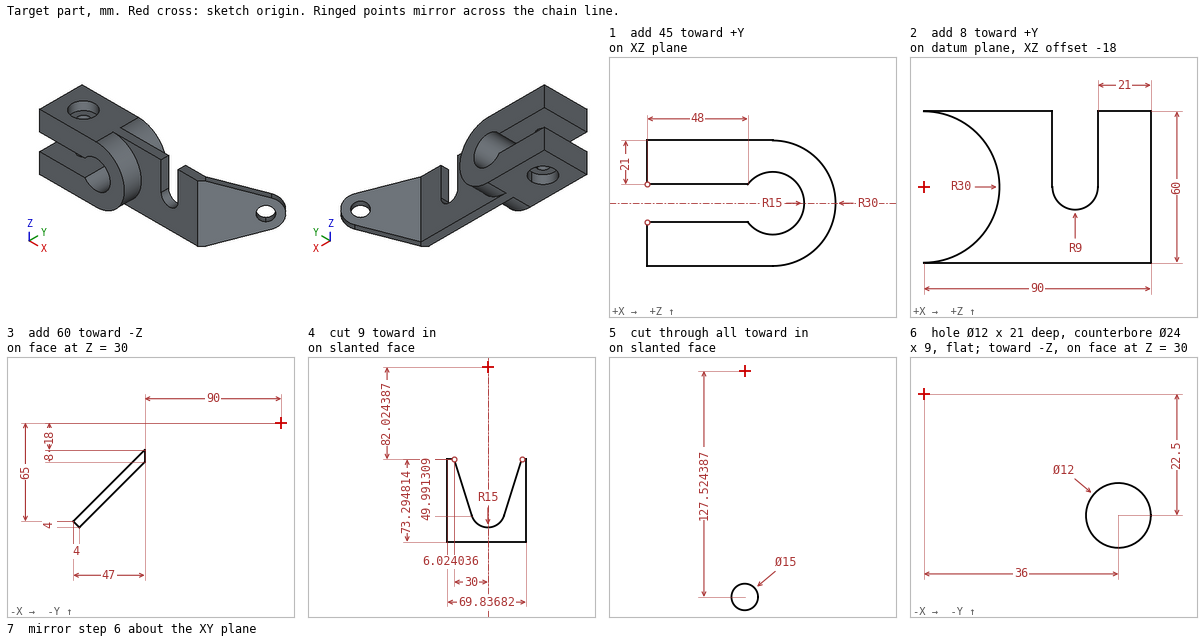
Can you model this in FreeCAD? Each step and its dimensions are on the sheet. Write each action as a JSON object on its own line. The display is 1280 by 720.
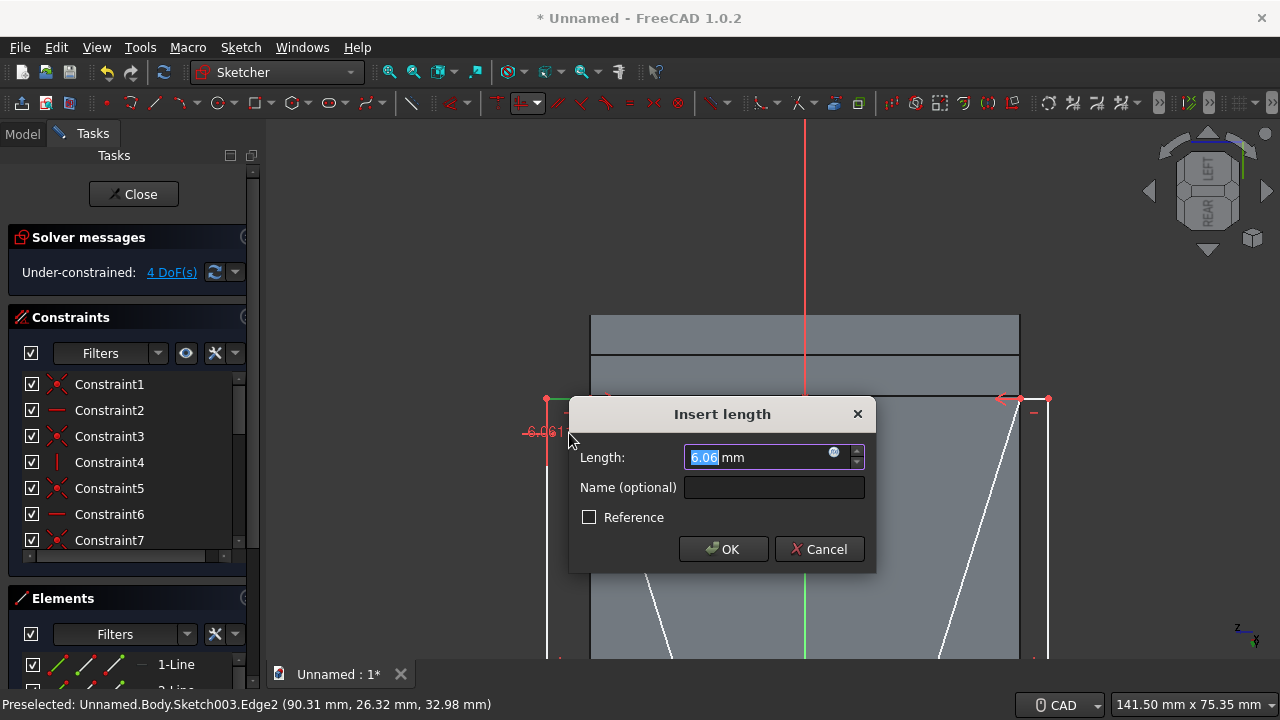
{"action": "type", "text": "6.024036"}
{"action": "key", "text": "Return"}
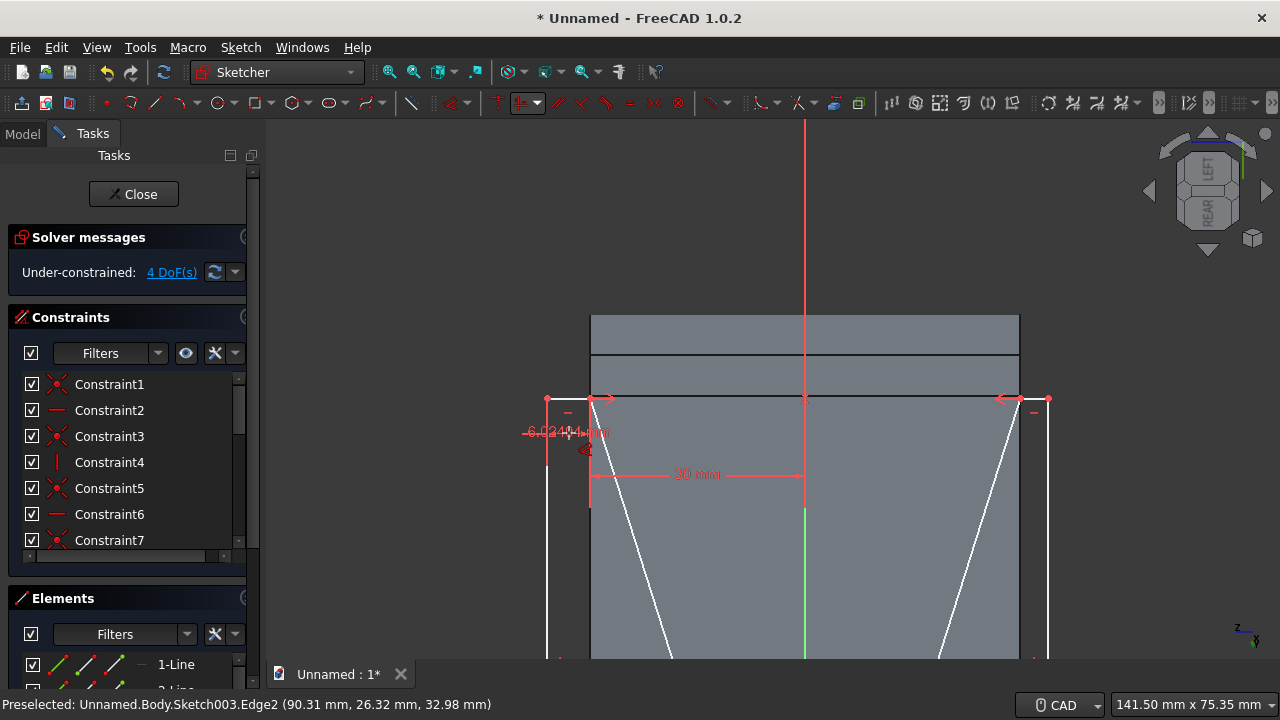
{"action": "scroll", "coordinate": [664, 400], "scroll_direction": "down", "scroll_amount": 6}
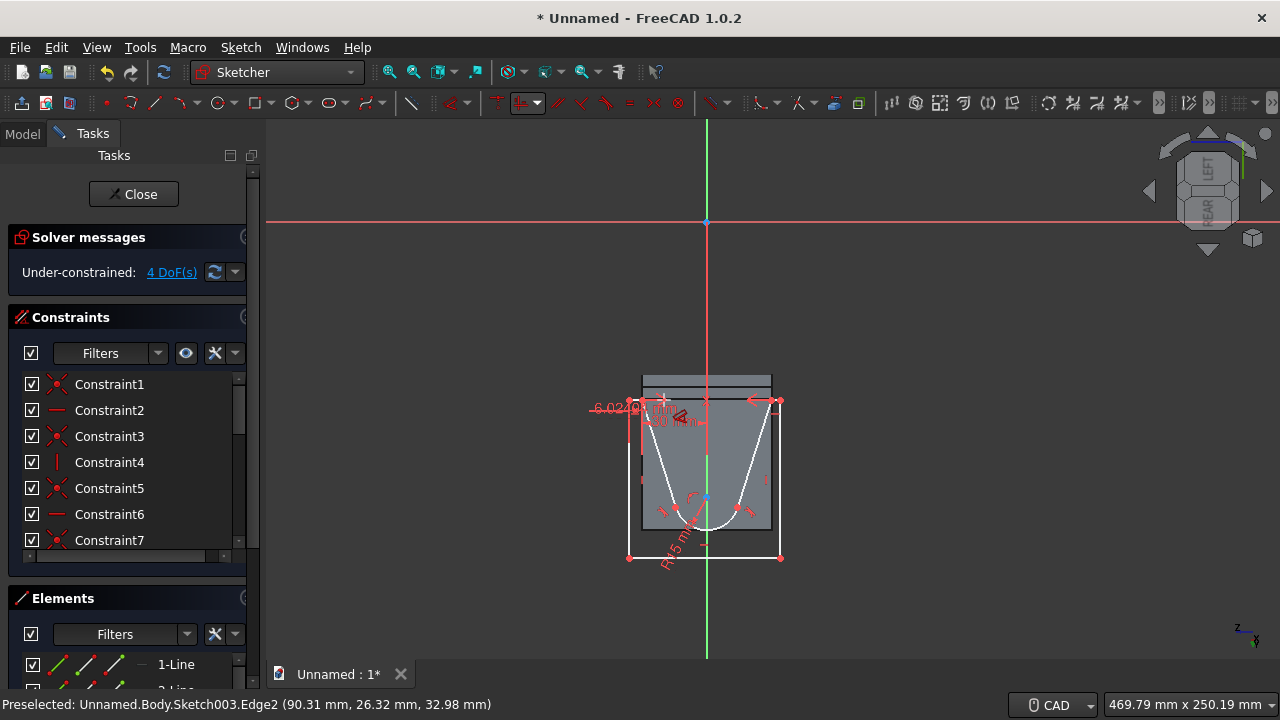
{"action": "left_click", "coordinate": [674, 558]}
{"action": "left_click", "coordinate": [670, 592]}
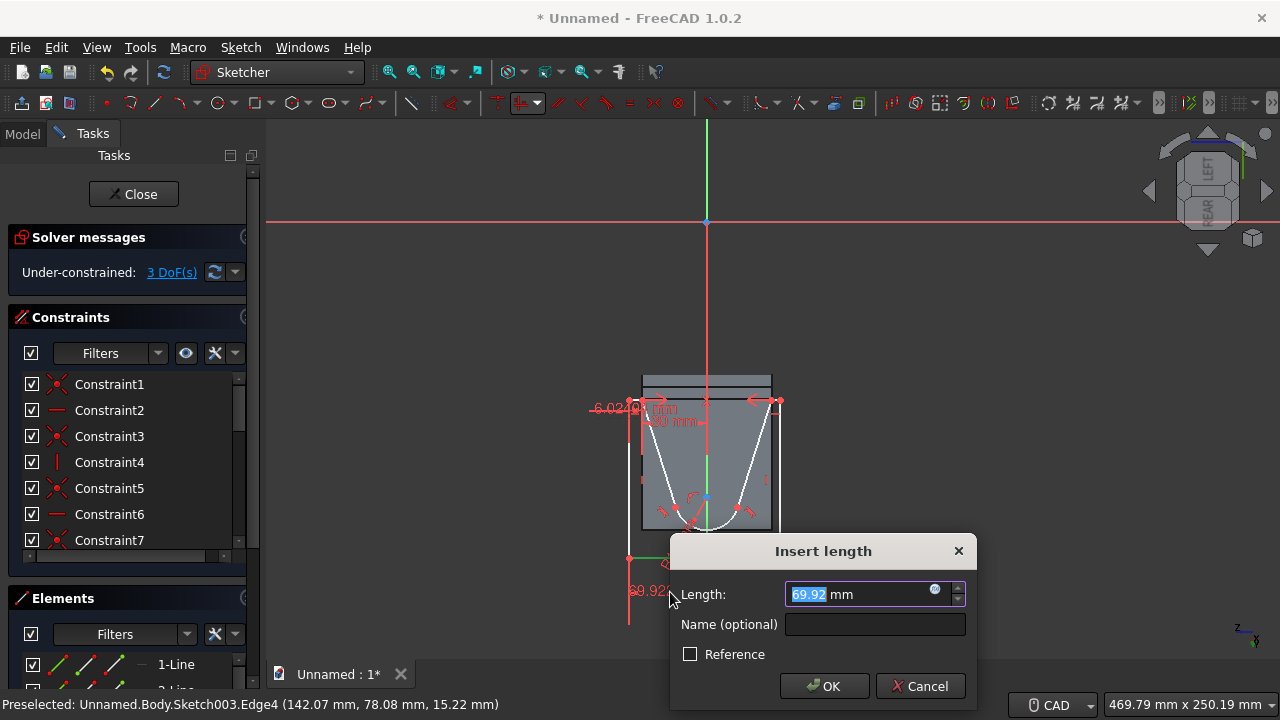
{"action": "type", "text": "69.83682"}
{"action": "key", "text": "Return"}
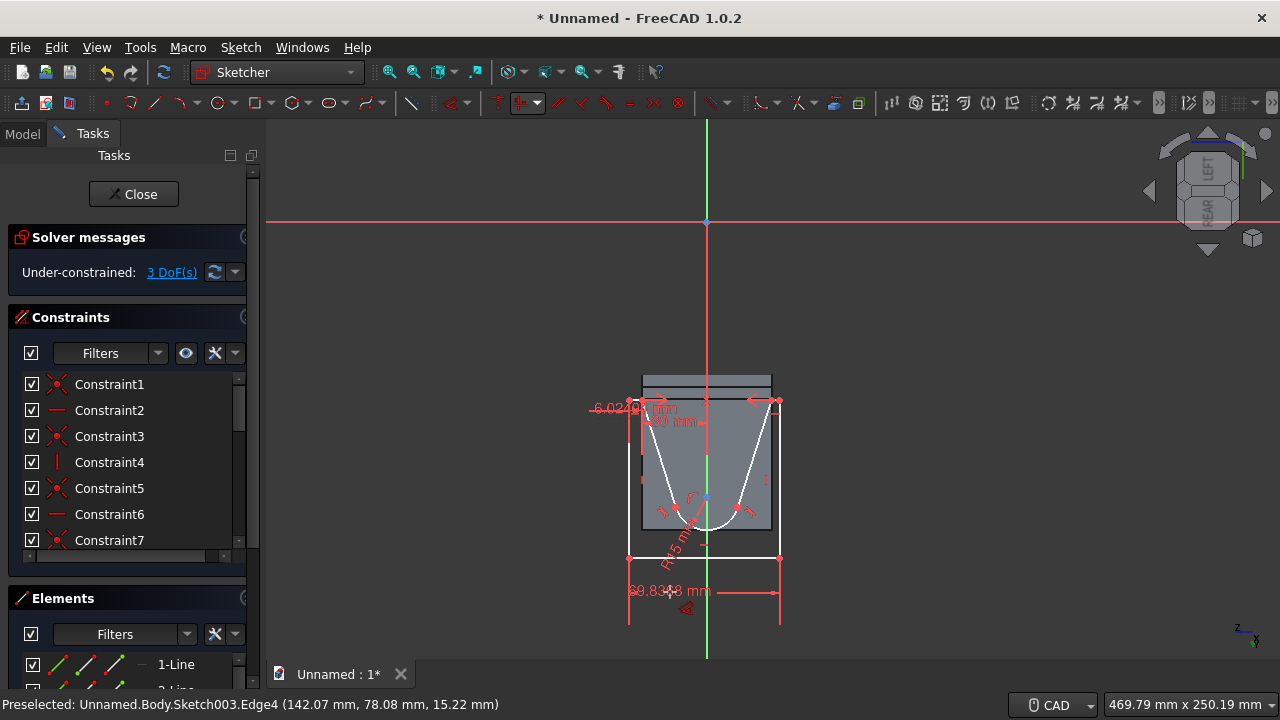
{"action": "left_click", "coordinate": [629, 447]}
{"action": "left_click", "coordinate": [595, 479]}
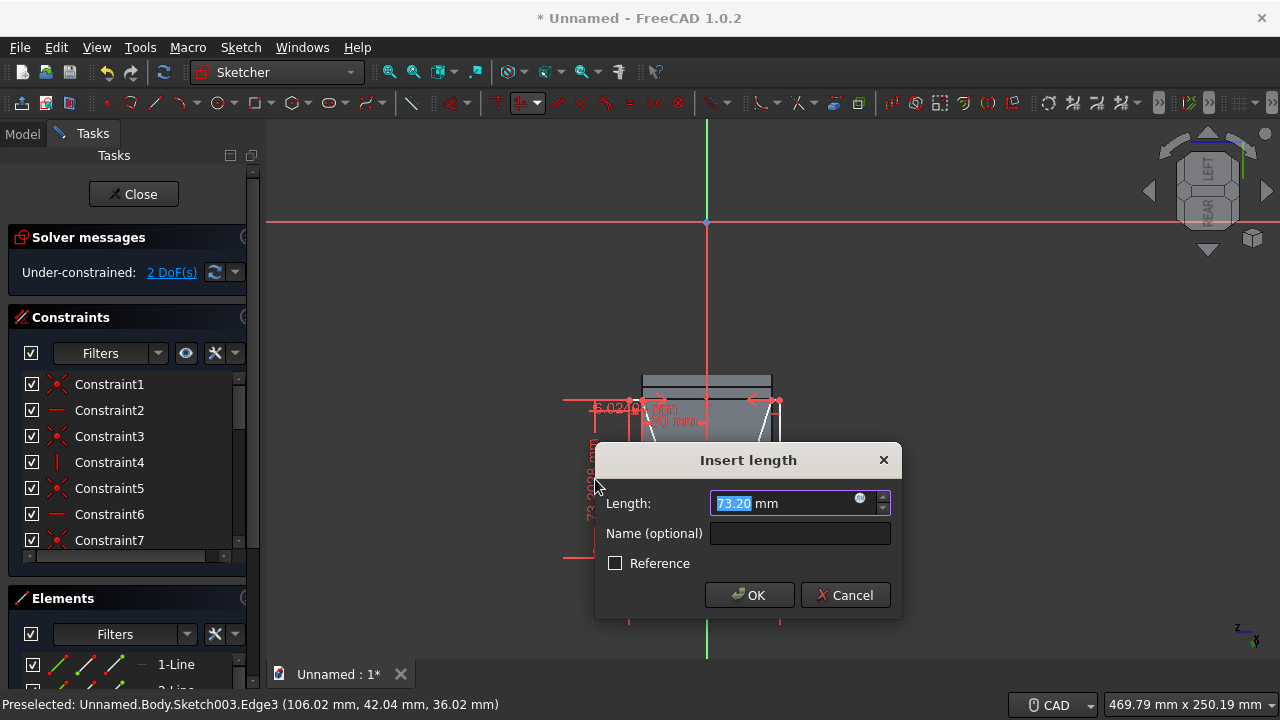
{"action": "type", "text": "73.294814"}
{"action": "key", "text": "Return"}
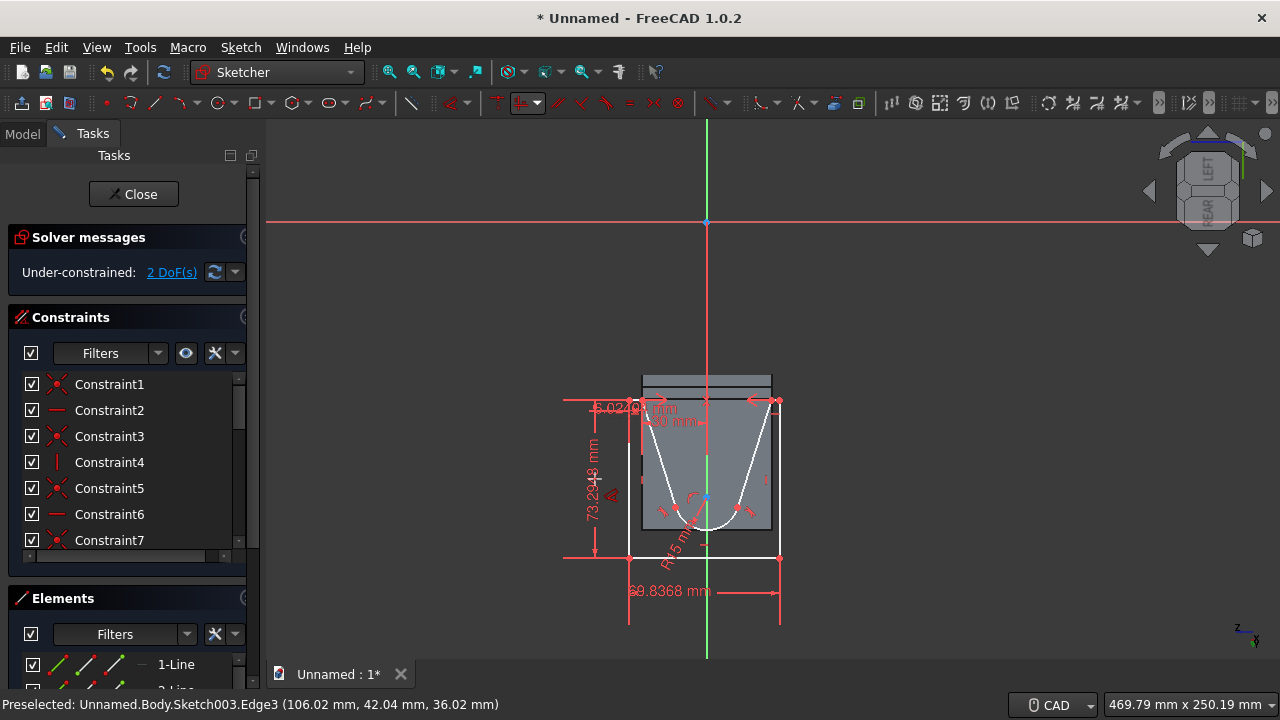
{"action": "left_click", "coordinate": [642, 400]}
{"action": "left_click", "coordinate": [608, 311]}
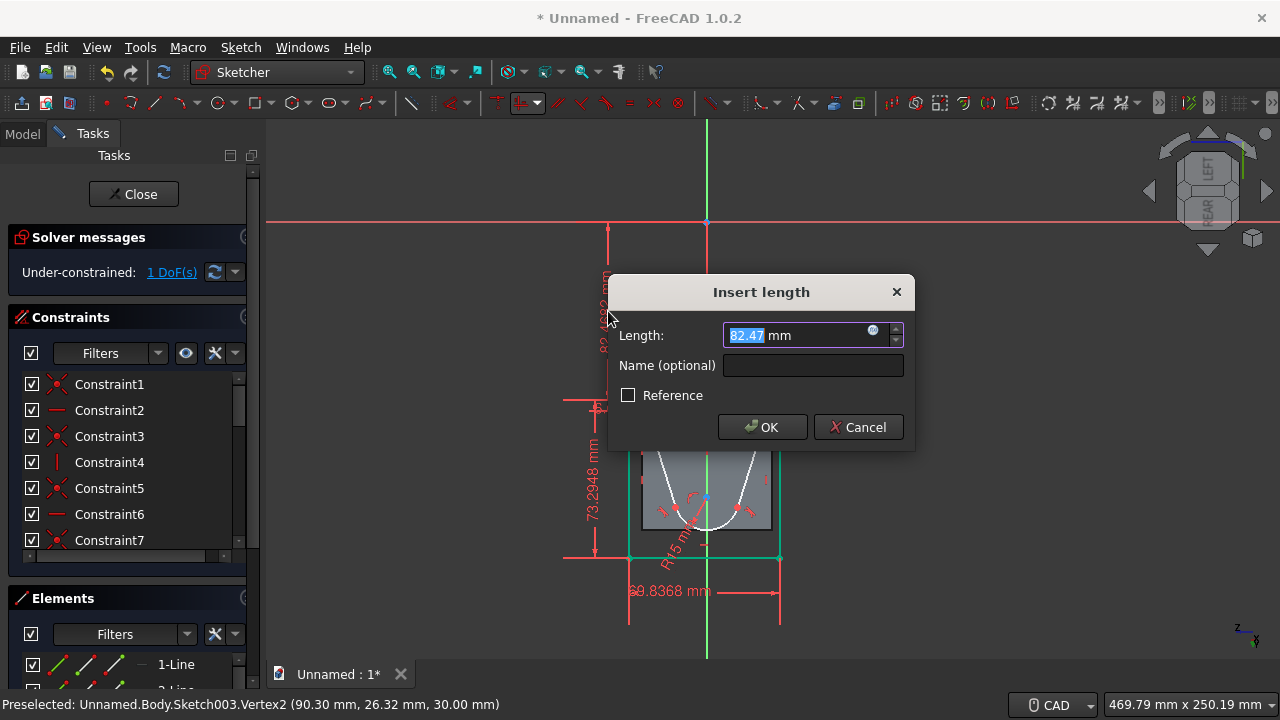
{"action": "type", "text": "82.024387"}
{"action": "key", "text": "Return"}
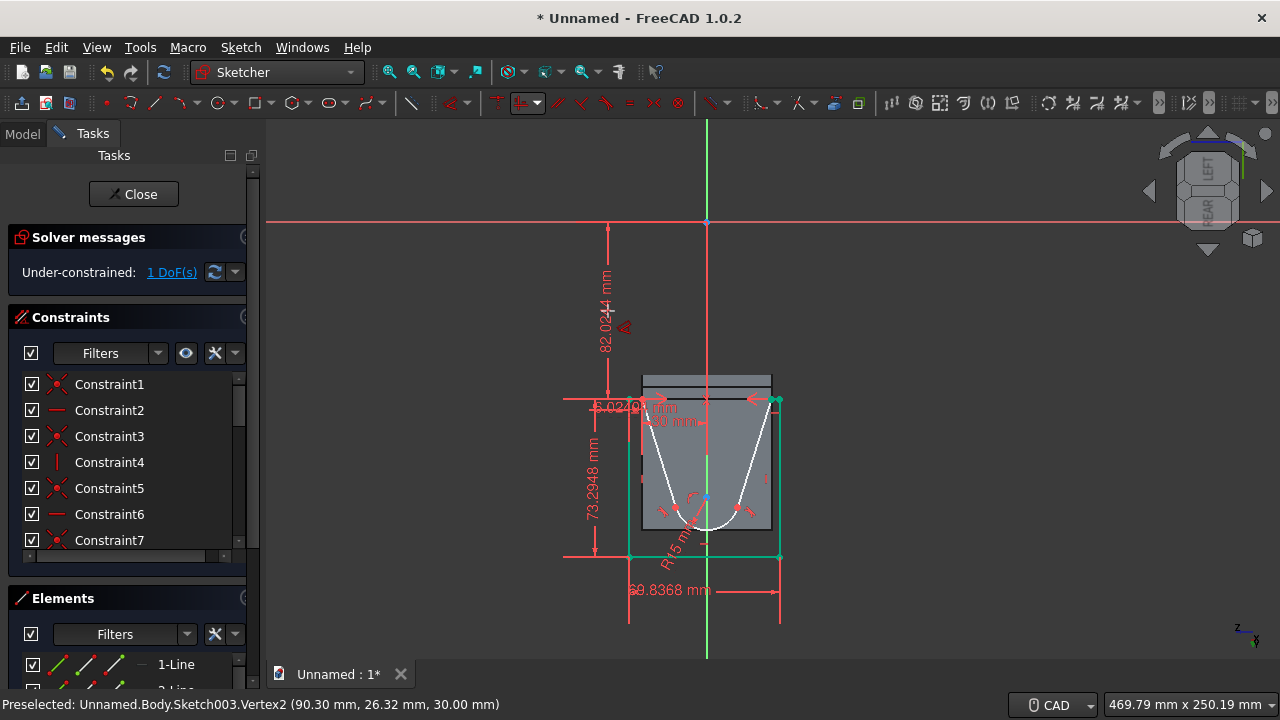
{"action": "left_click", "coordinate": [666, 475]}
{"action": "left_click", "coordinate": [608, 453]}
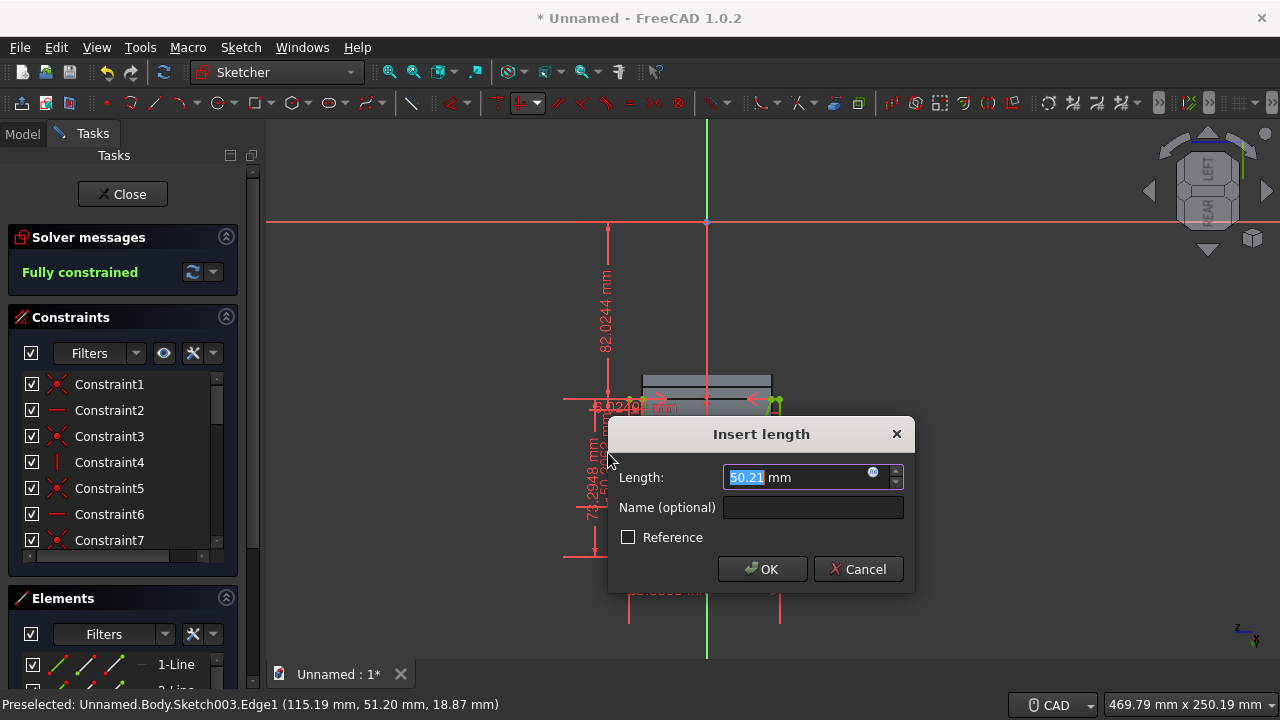
{"action": "type", "text": "49.991309"}
{"action": "key", "text": "Return"}
{"action": "key", "text": "Escape"}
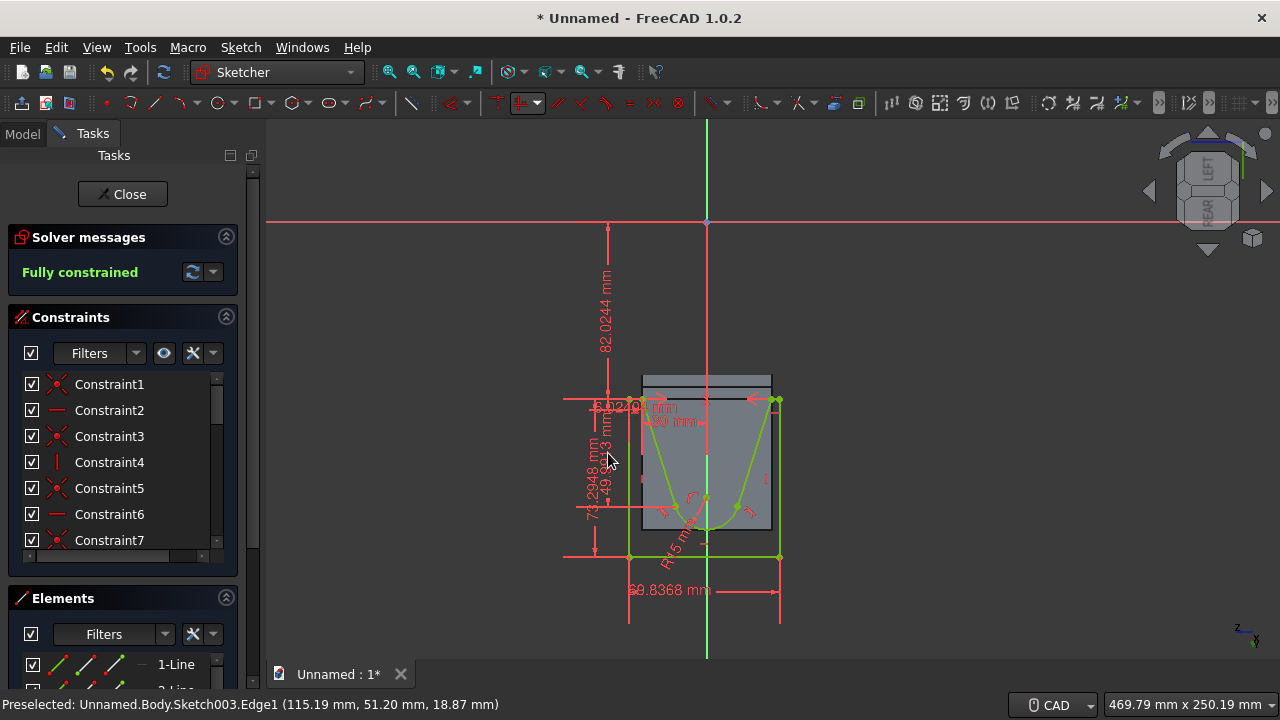
{"action": "left_click", "coordinate": [123, 194]}